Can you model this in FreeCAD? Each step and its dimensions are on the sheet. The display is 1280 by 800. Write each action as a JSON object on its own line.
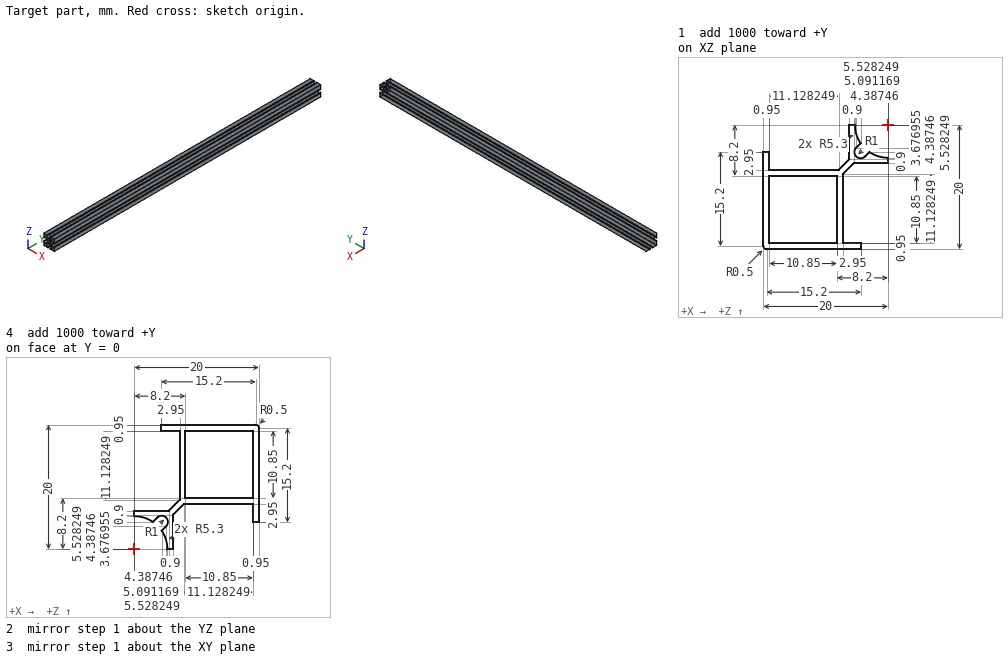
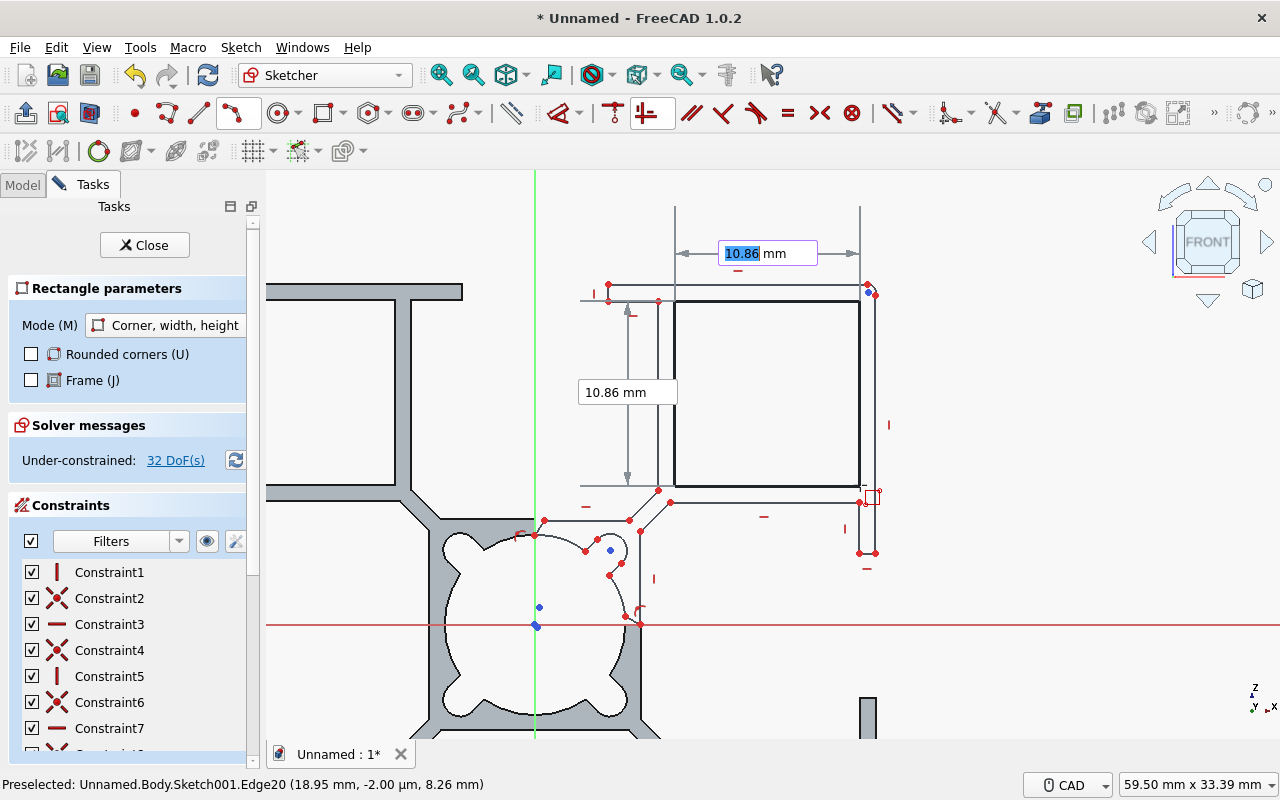
{"action": "type", "text": "10.85"}
{"action": "key", "text": "Tab"}
{"action": "type", "text": "10.85"}
{"action": "key", "text": "Return"}
{"action": "key", "text": "Escape"}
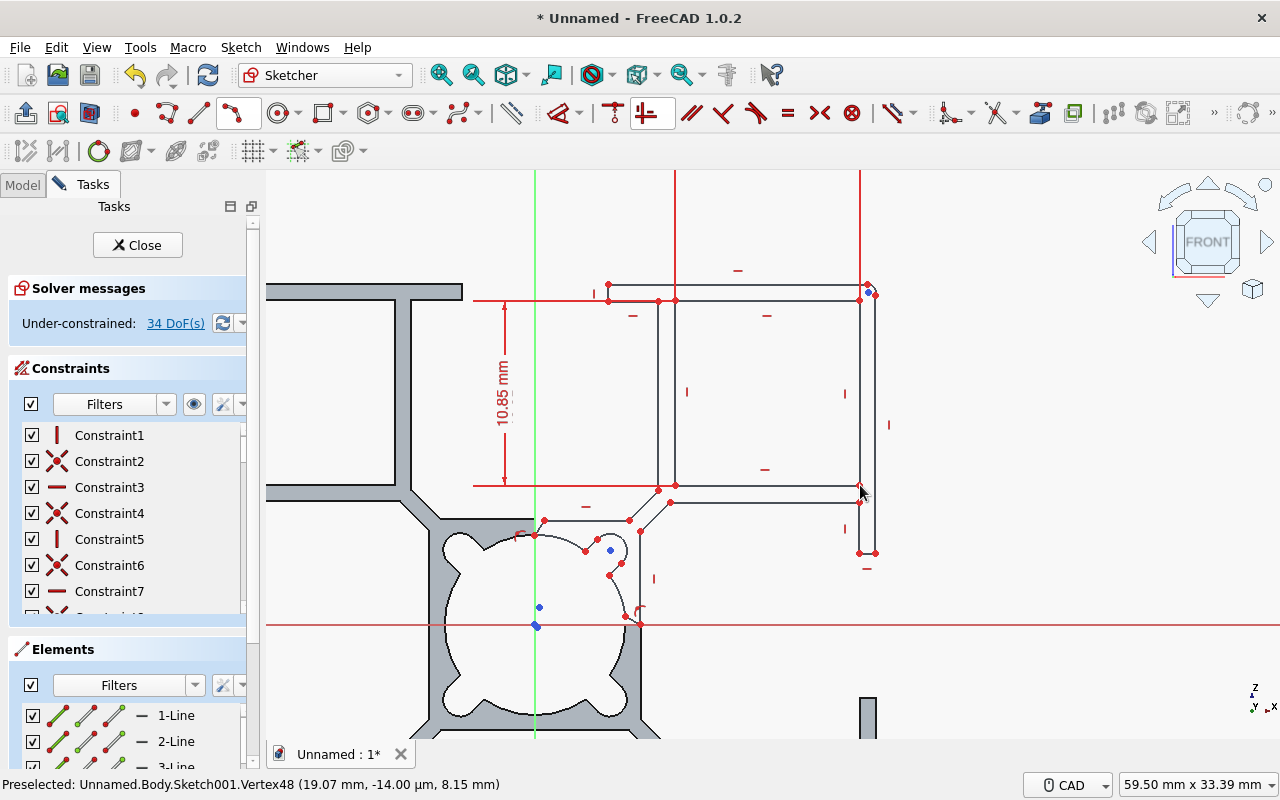
{"action": "left_click", "coordinate": [875, 373]}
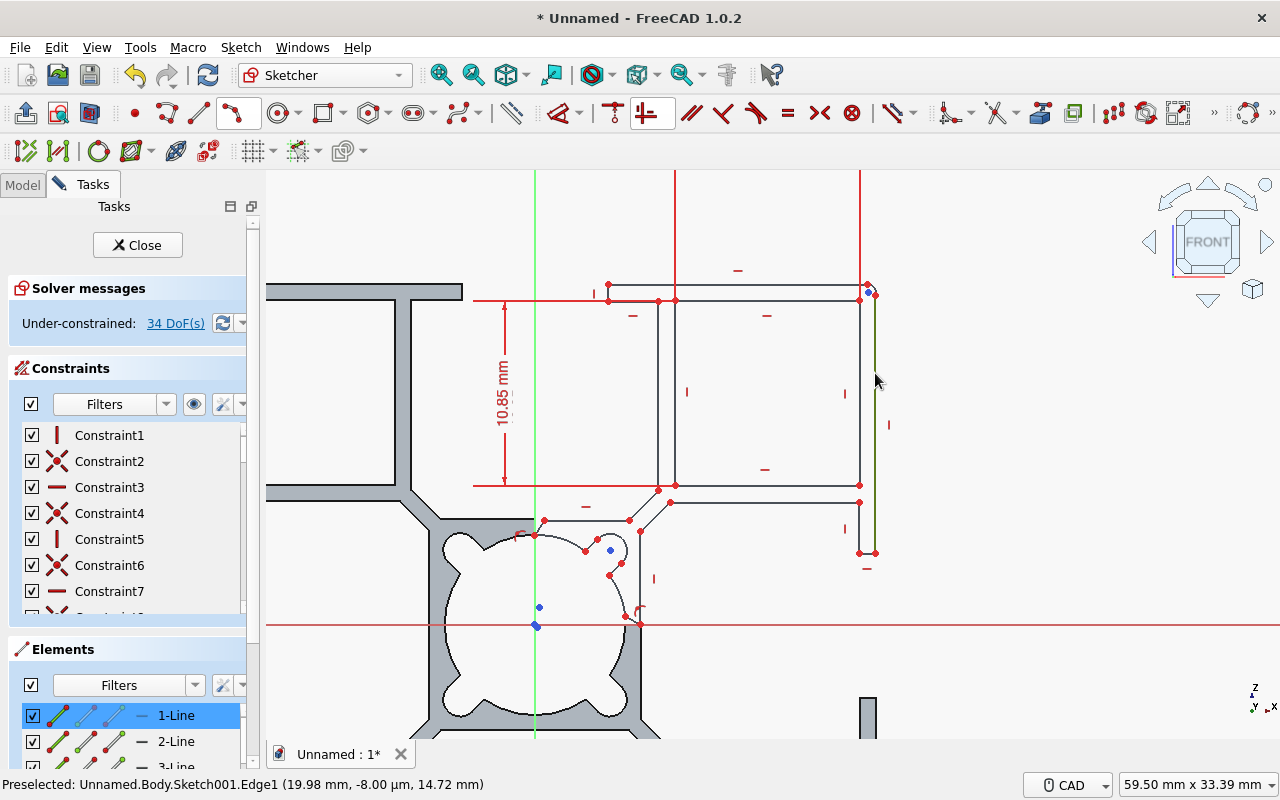
{"action": "scroll", "coordinate": [874, 288], "scroll_direction": "up", "scroll_amount": 4}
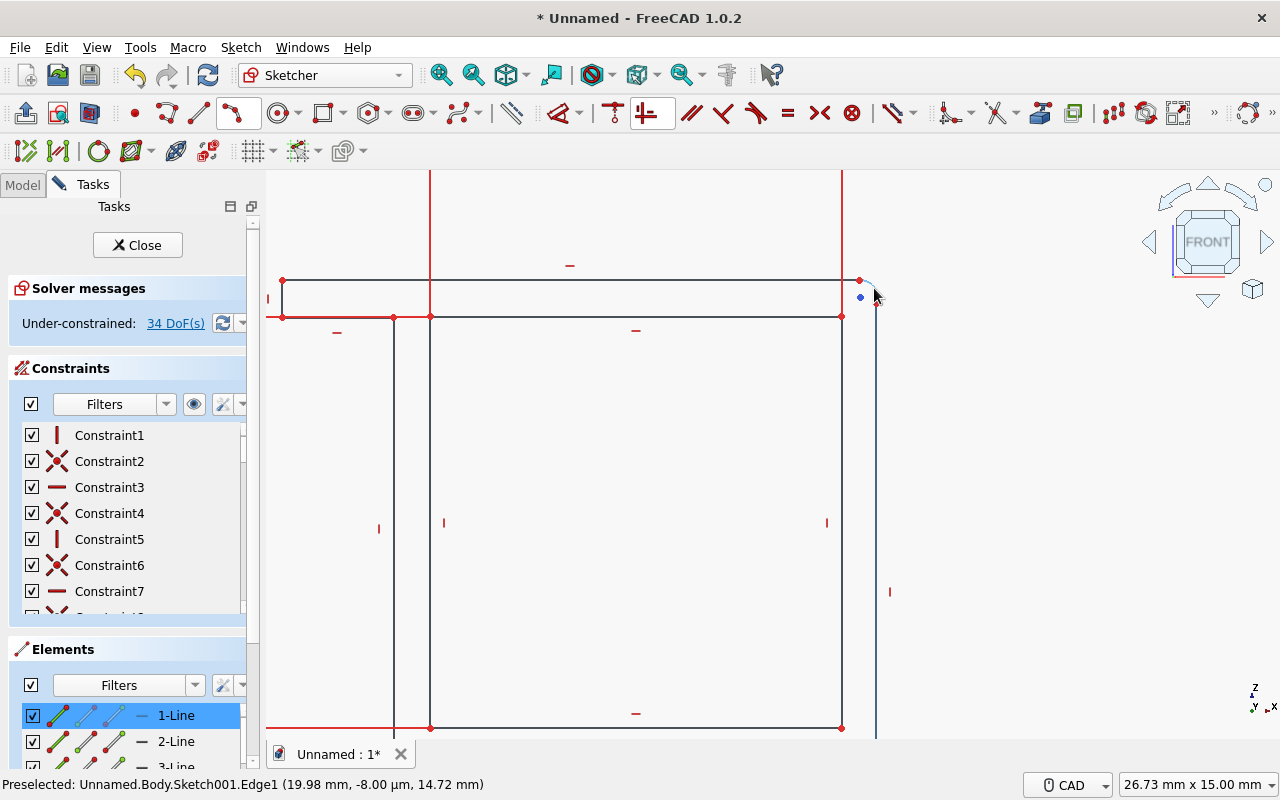
{"action": "left_click", "coordinate": [874, 287]}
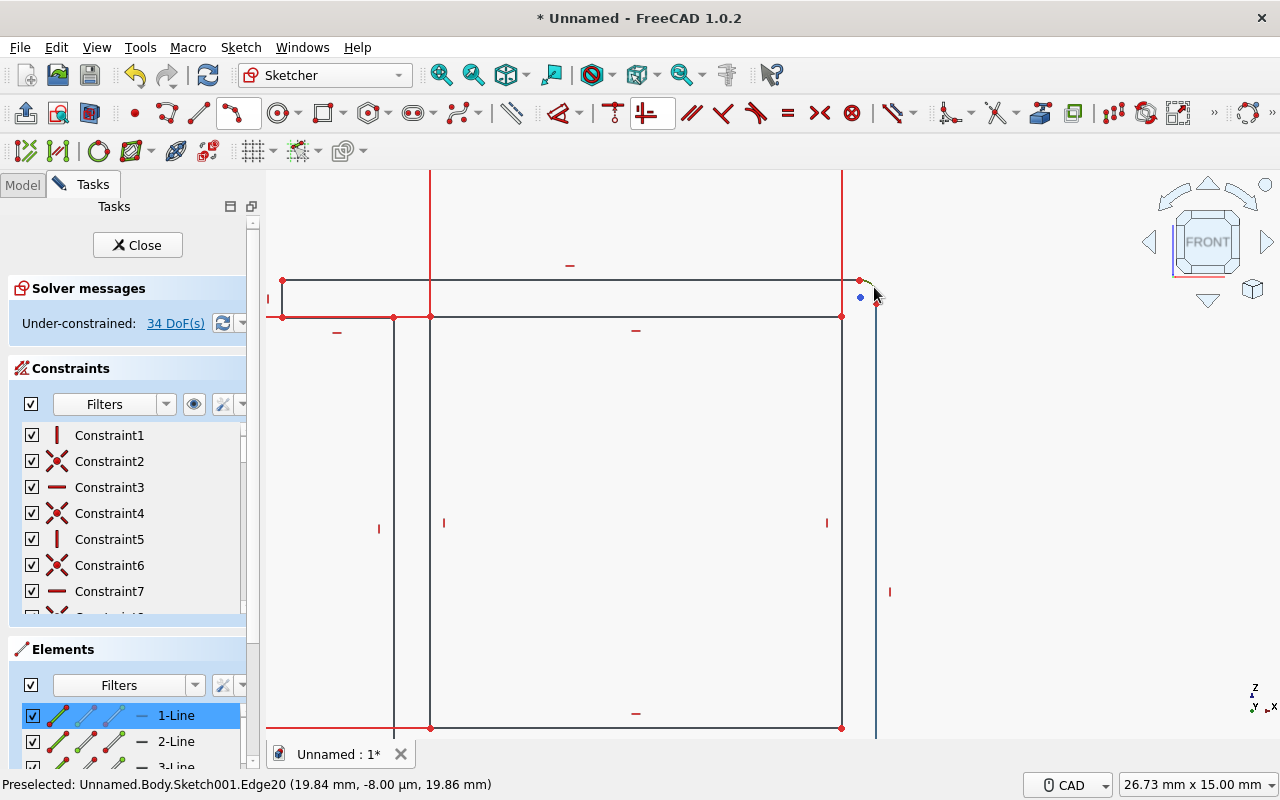
{"action": "left_click", "coordinate": [756, 114]}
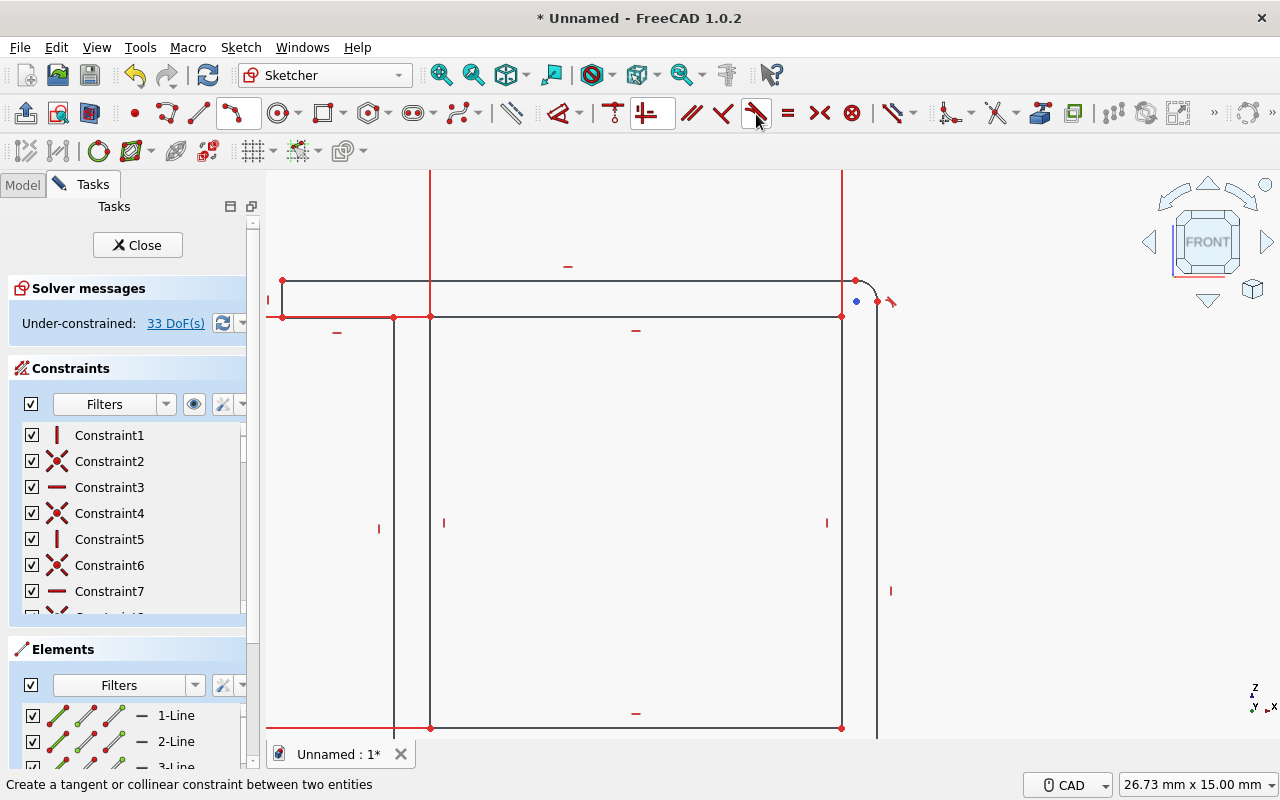
{"action": "scroll", "coordinate": [873, 288], "scroll_direction": "down", "scroll_amount": 4}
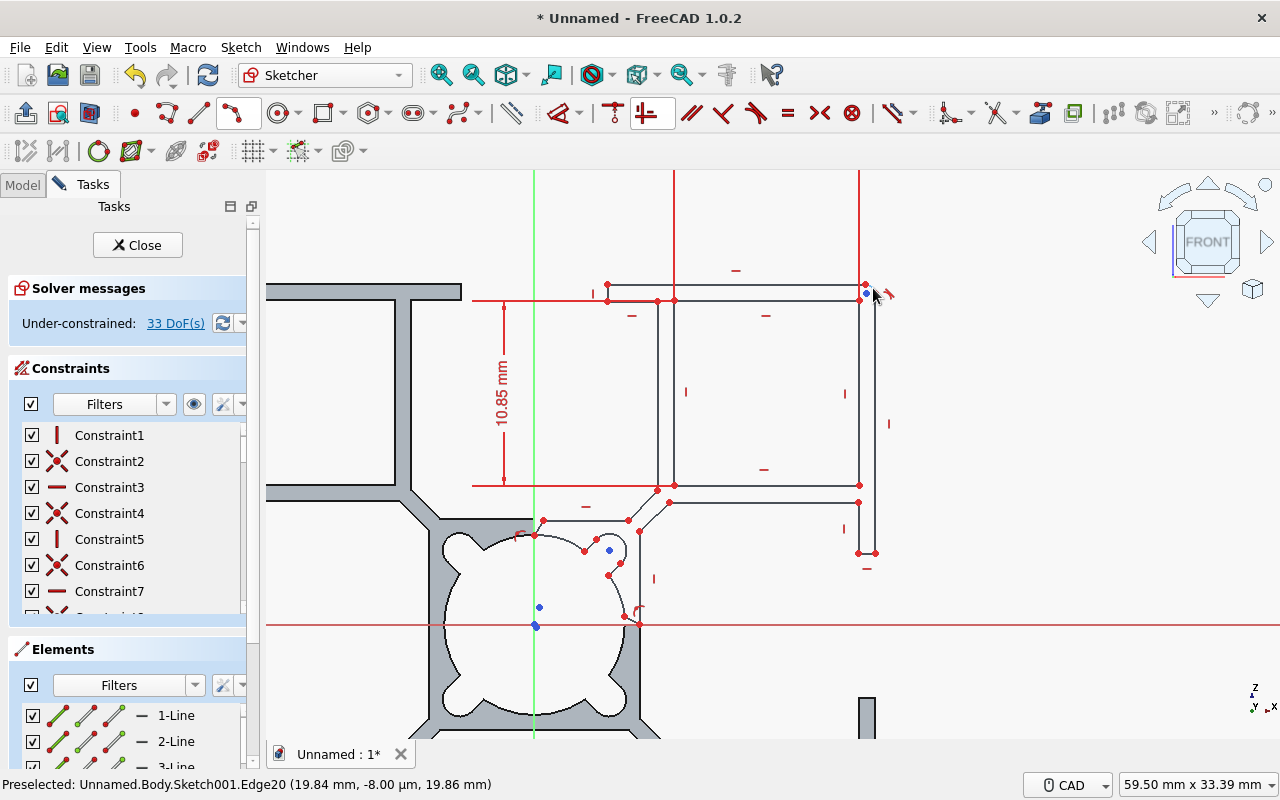
{"action": "scroll", "coordinate": [612, 572], "scroll_direction": "up", "scroll_amount": 5}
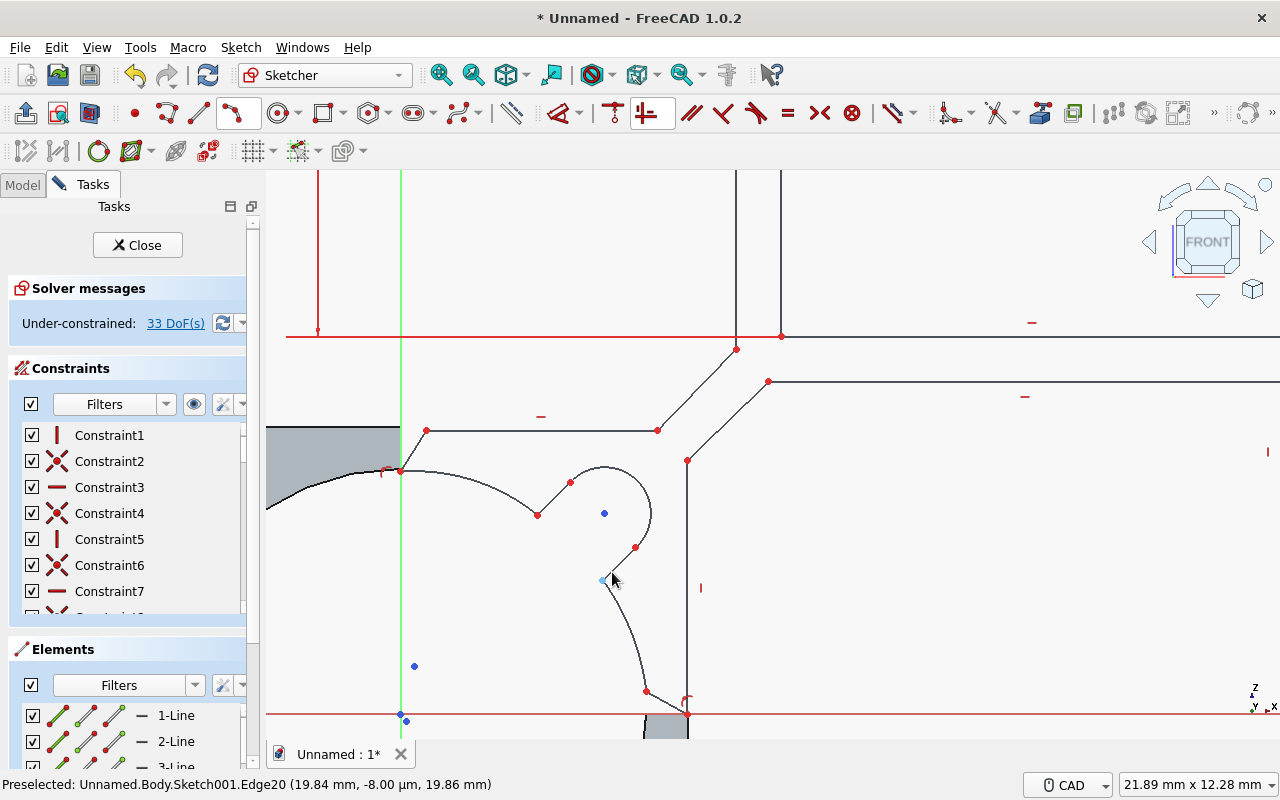
{"action": "left_click", "coordinate": [613, 571]}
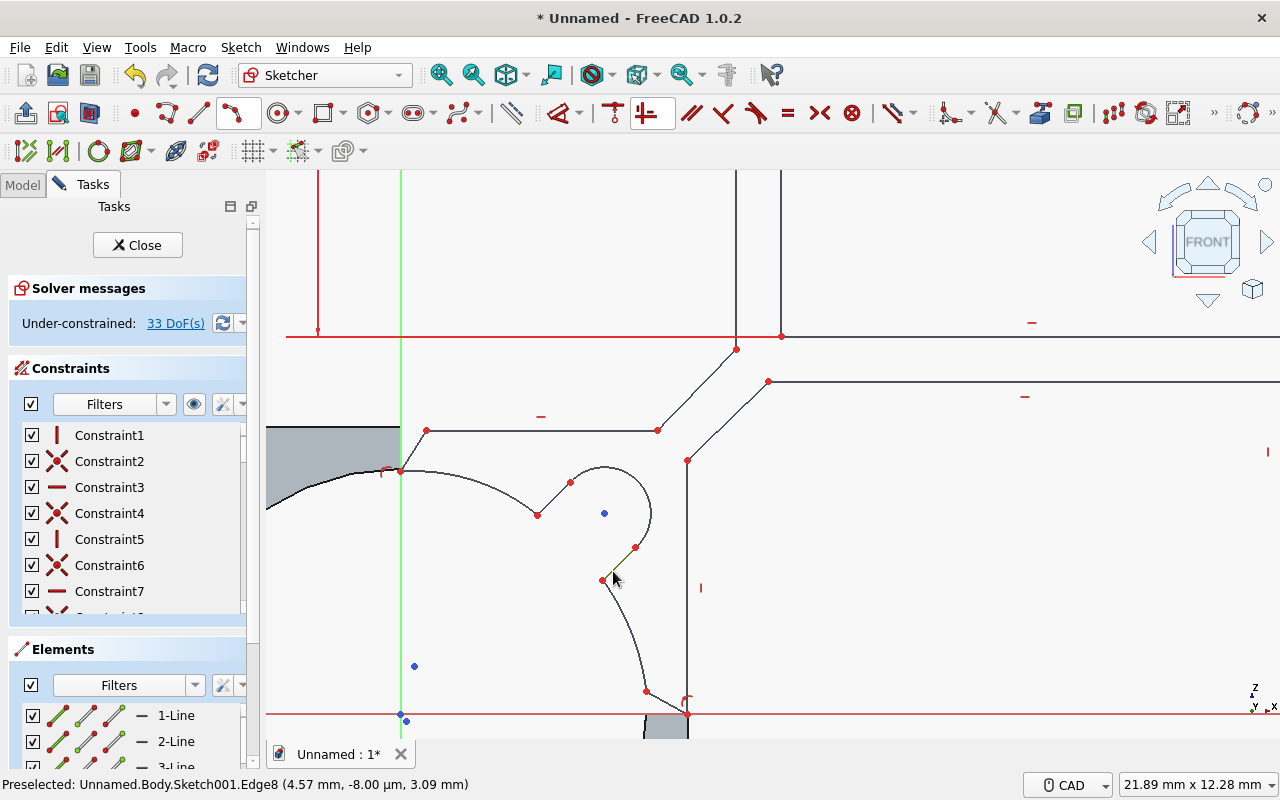
{"action": "left_click", "coordinate": [650, 507]}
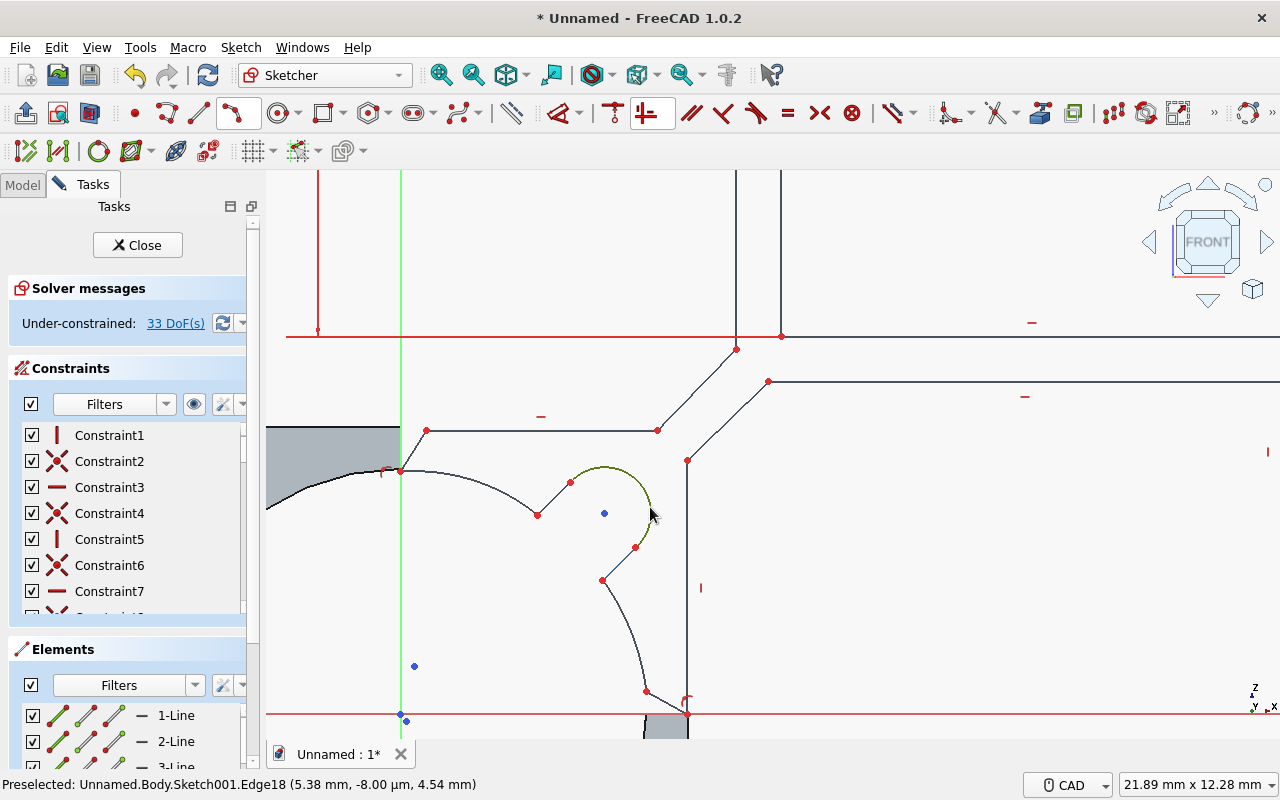
{"action": "left_click", "coordinate": [756, 114]}